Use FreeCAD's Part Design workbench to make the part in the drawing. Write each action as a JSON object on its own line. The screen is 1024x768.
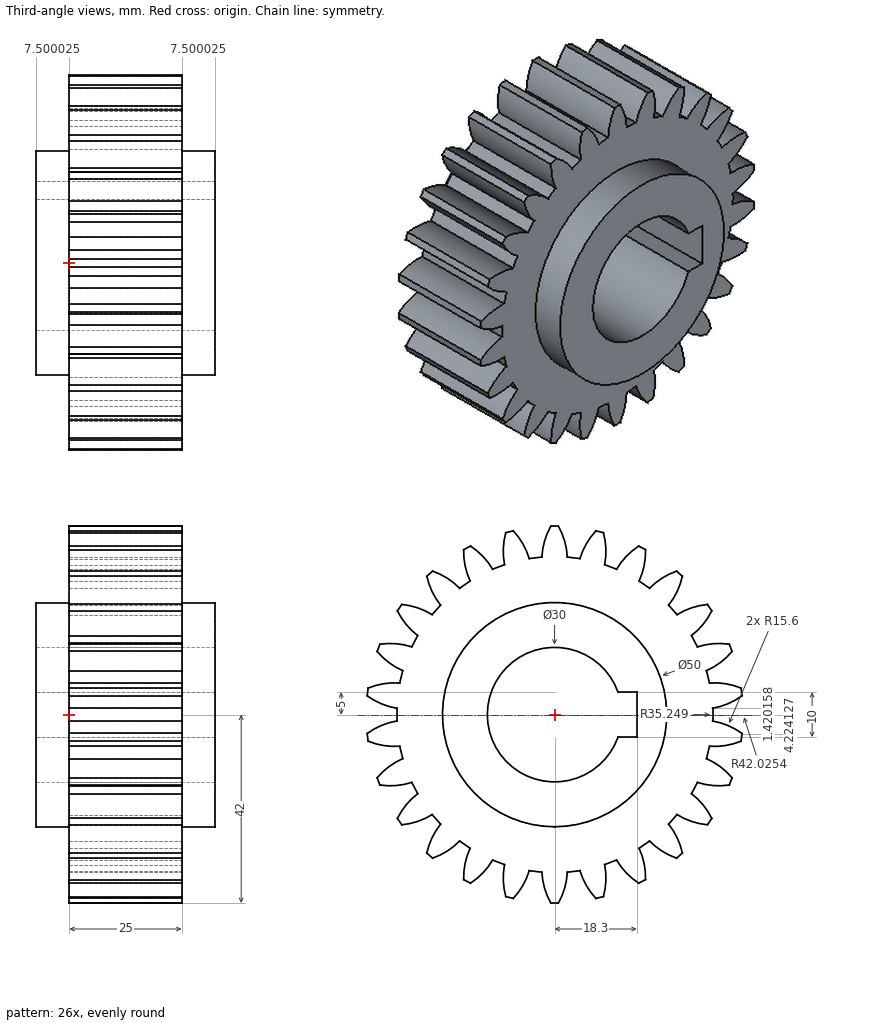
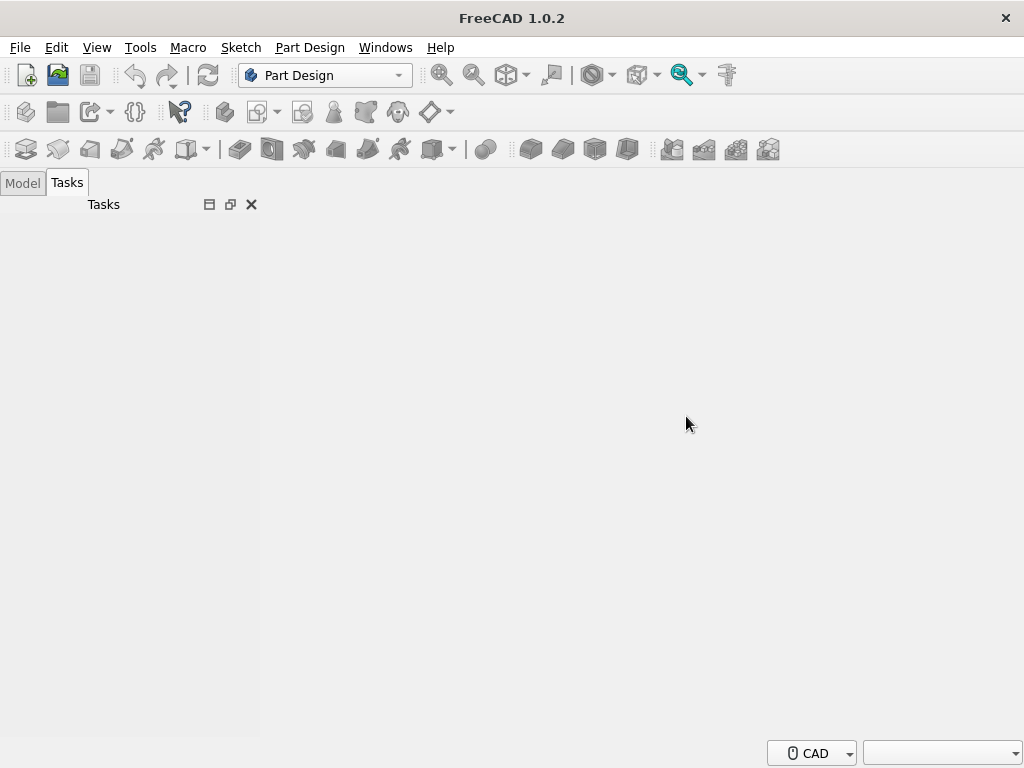
{"action": "left_click", "coordinate": [26, 76]}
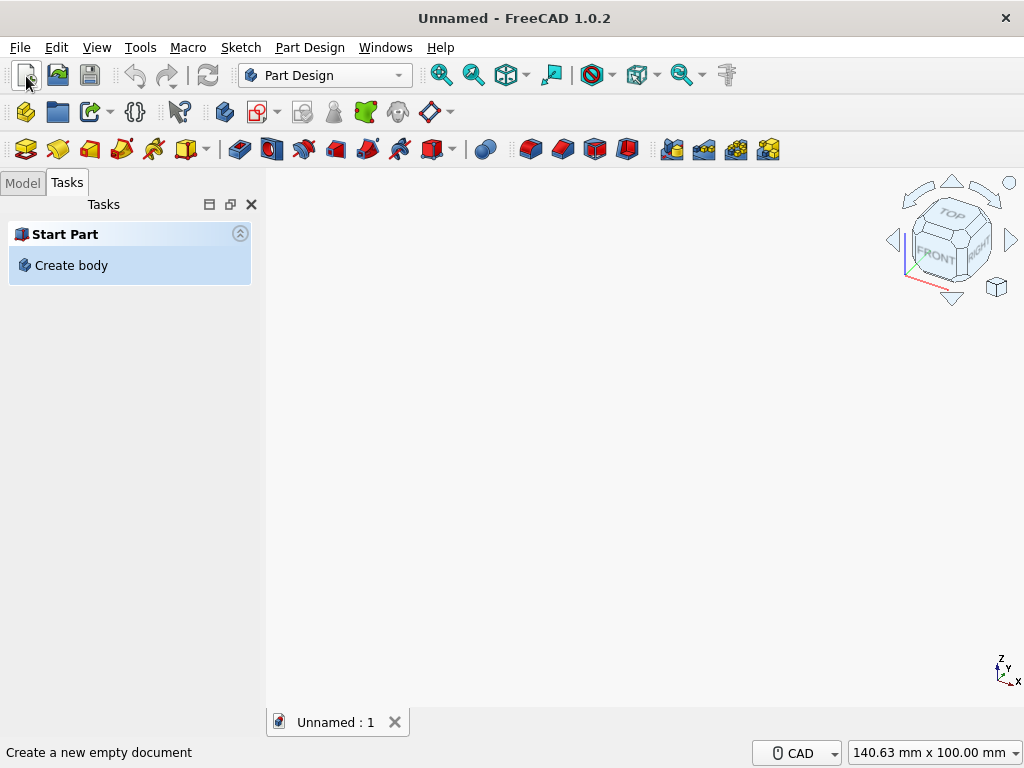
{"action": "left_click", "coordinate": [258, 112]}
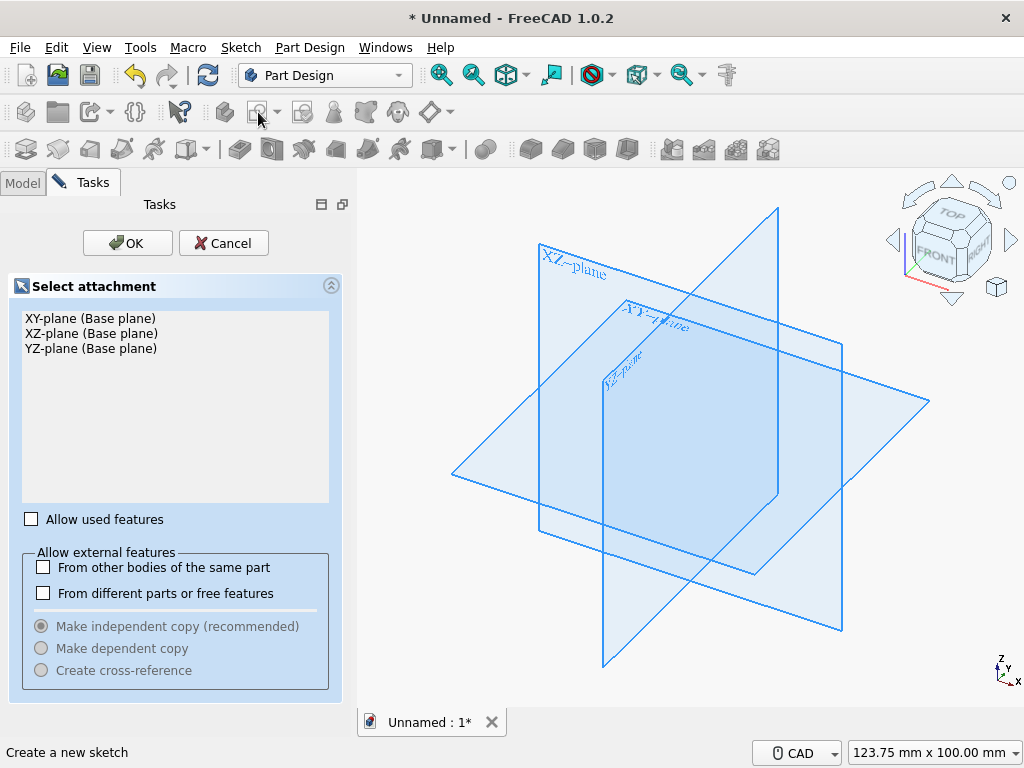
{"action": "left_click", "coordinate": [82, 334]}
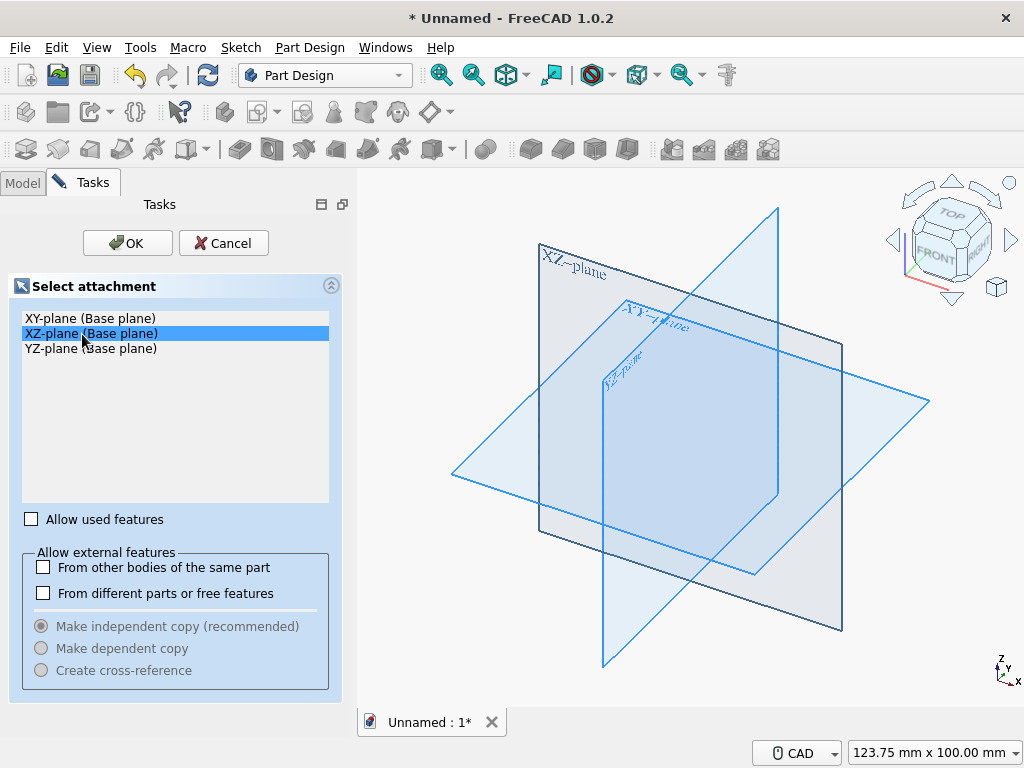
{"action": "left_click", "coordinate": [128, 243]}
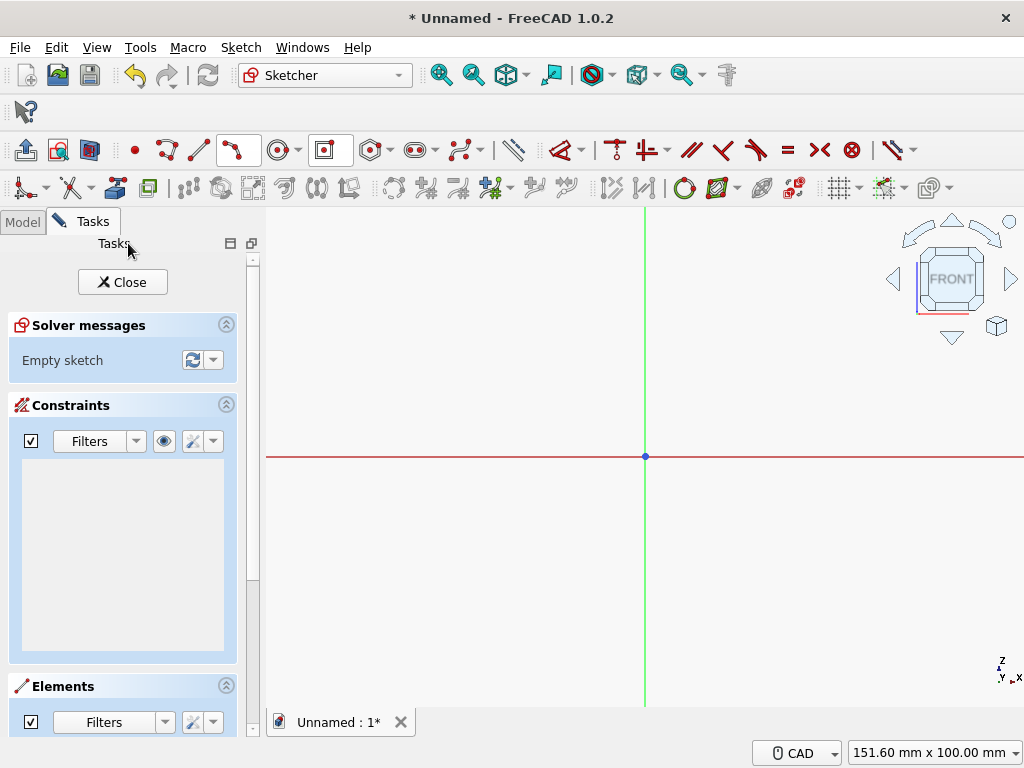
{"action": "scroll", "coordinate": [294, 235], "scroll_direction": "down", "scroll_amount": 1}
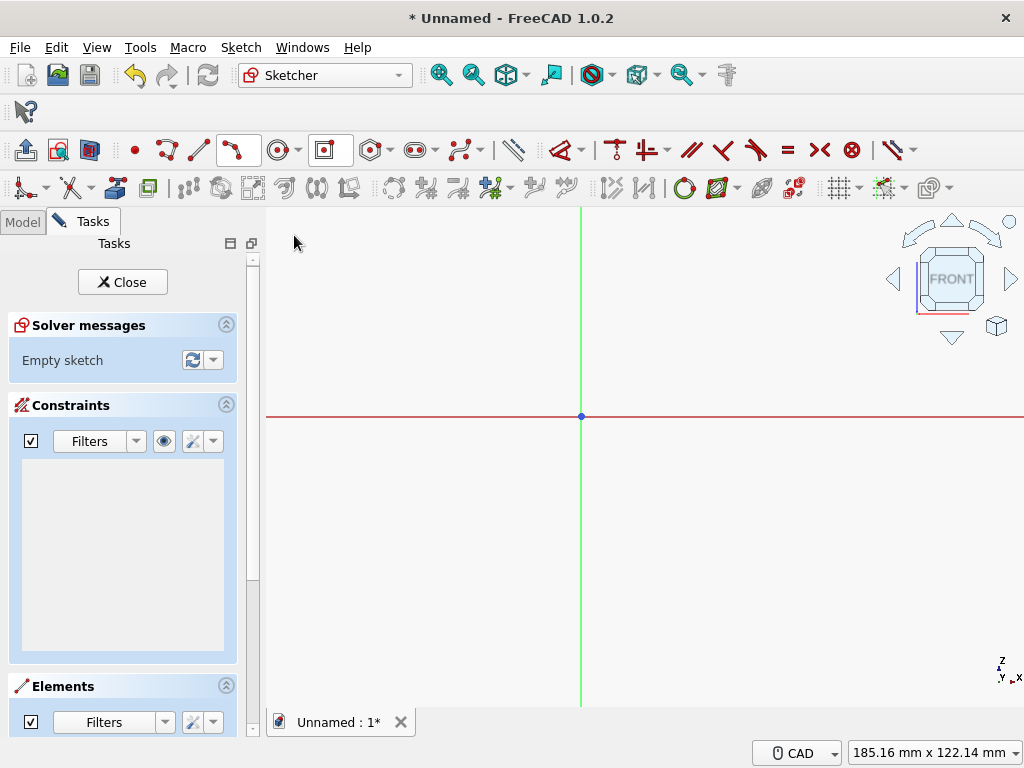
{"action": "scroll", "coordinate": [701, 558], "scroll_direction": "up", "scroll_amount": 3}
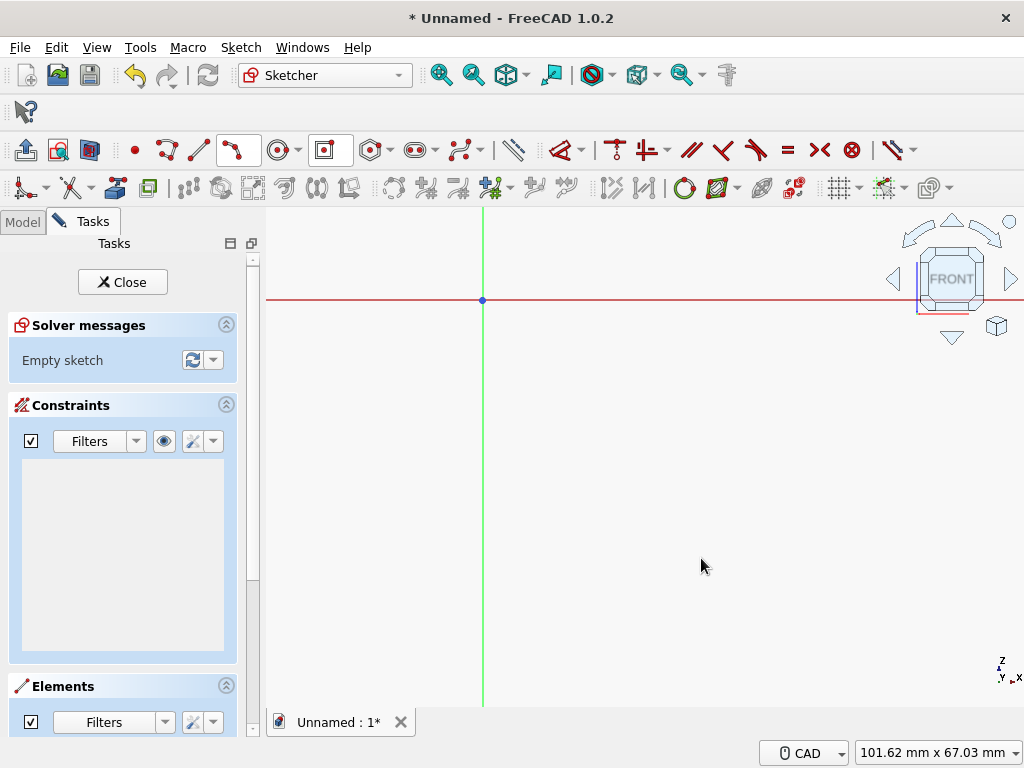
{"action": "left_click", "coordinate": [348, 150]}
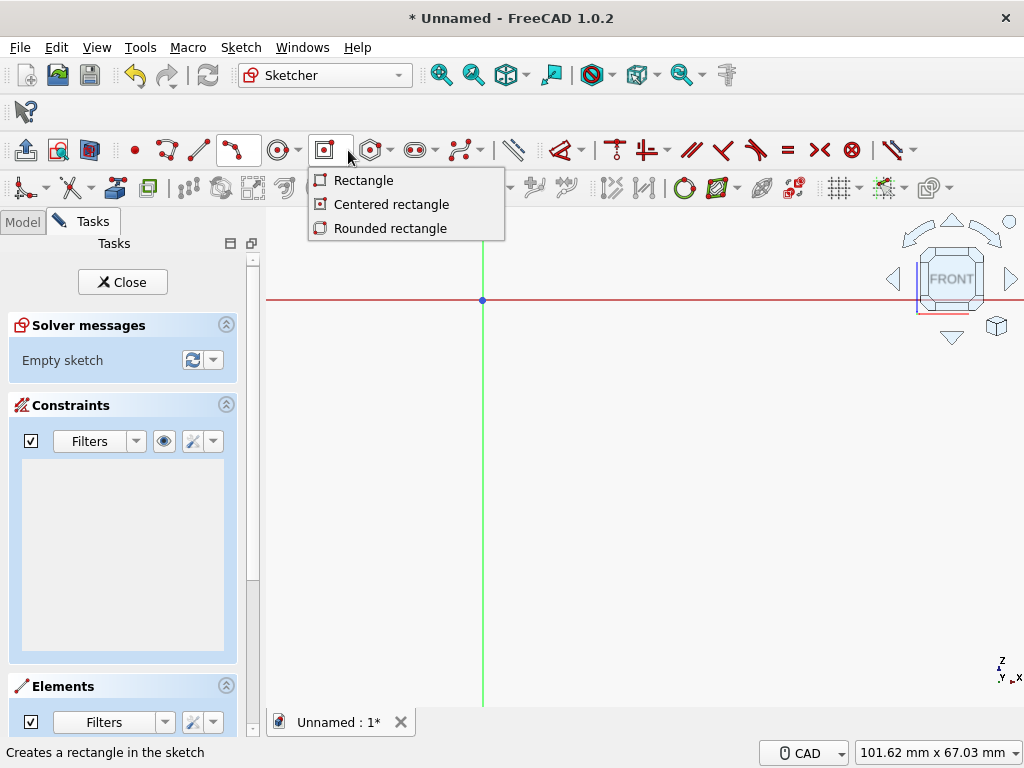
{"action": "left_click", "coordinate": [406, 180]}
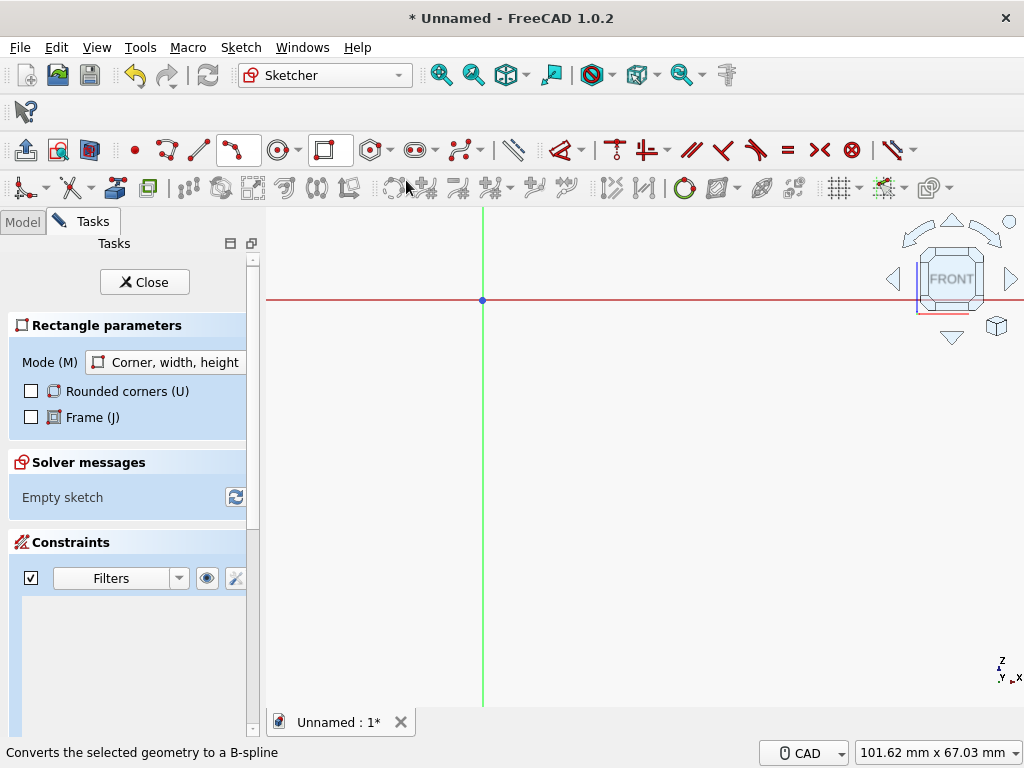
{"action": "left_click", "coordinate": [483, 300]}
{"action": "mouse_move", "coordinate": [669, 613]}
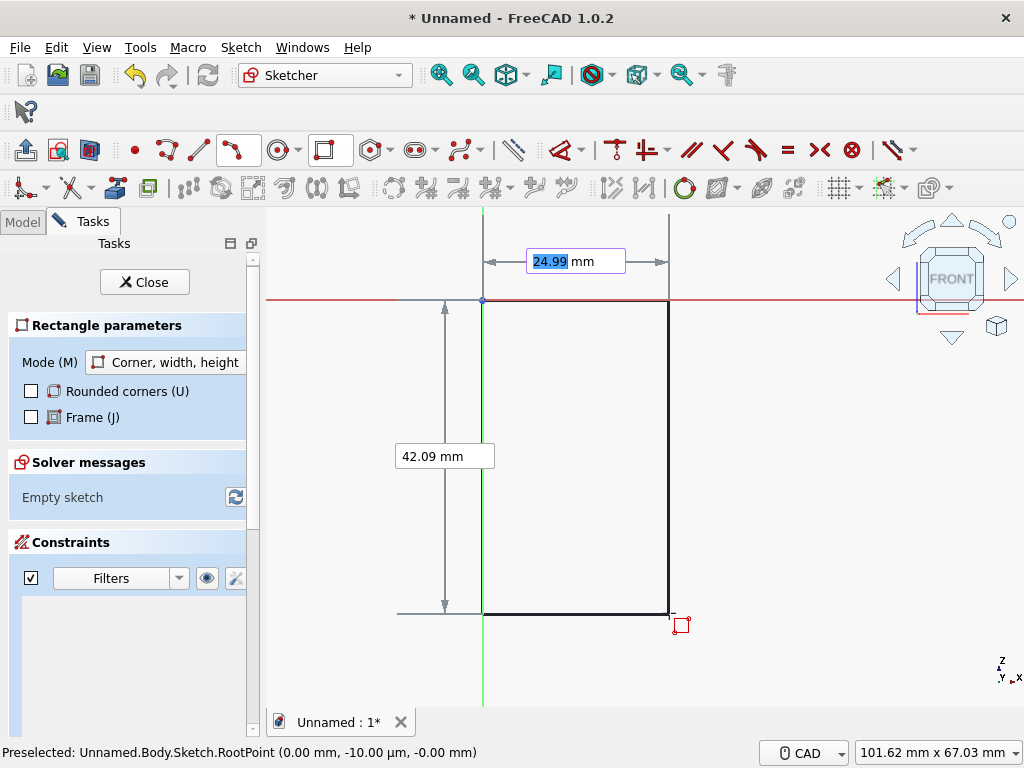
{"action": "type", "text": "25"}
{"action": "key", "text": "Tab"}
{"action": "type", "text": "42"}
{"action": "key", "text": "Return"}
{"action": "key", "text": "Escape"}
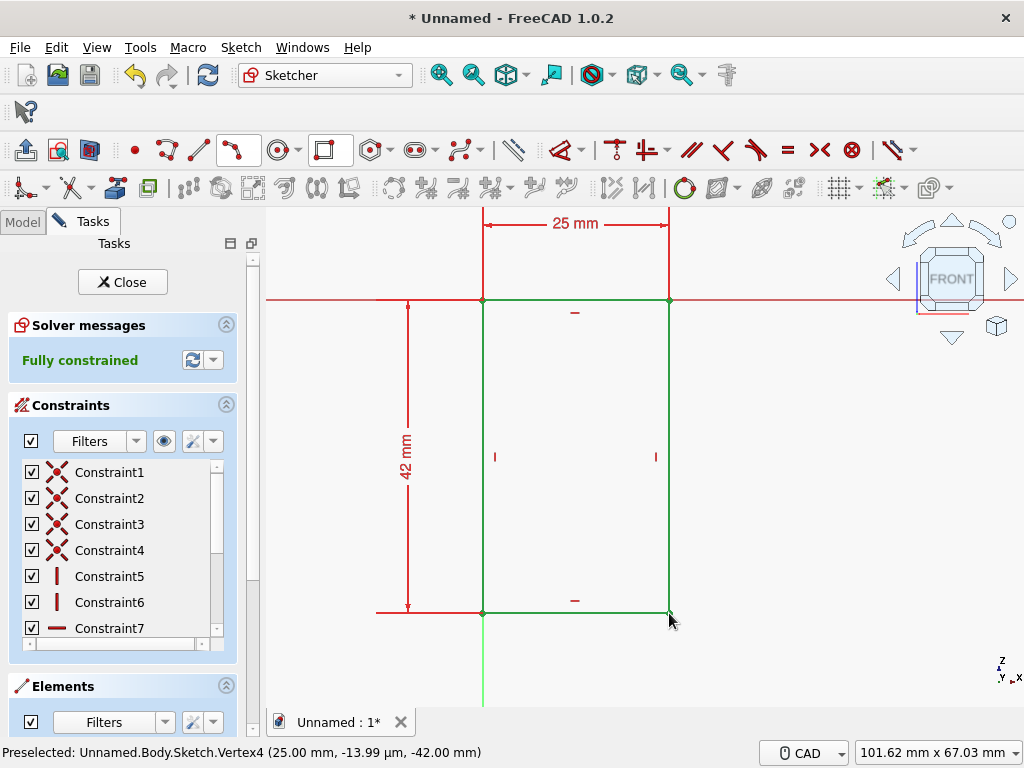
{"action": "left_click", "coordinate": [123, 282]}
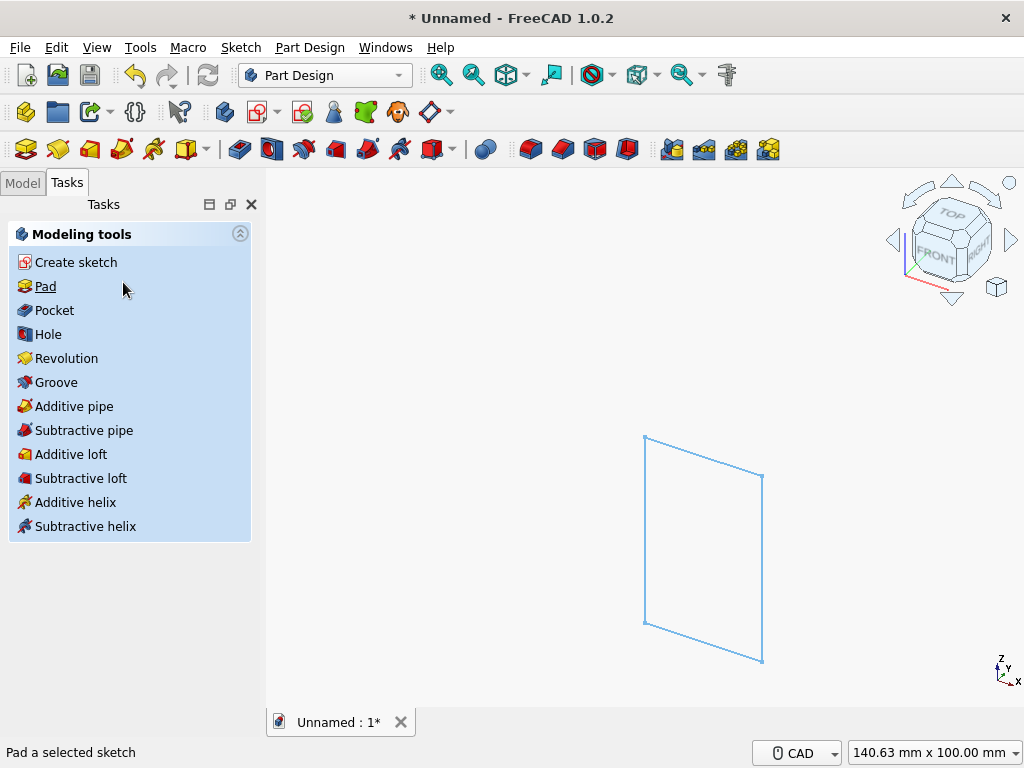
{"action": "left_click", "coordinate": [58, 150]}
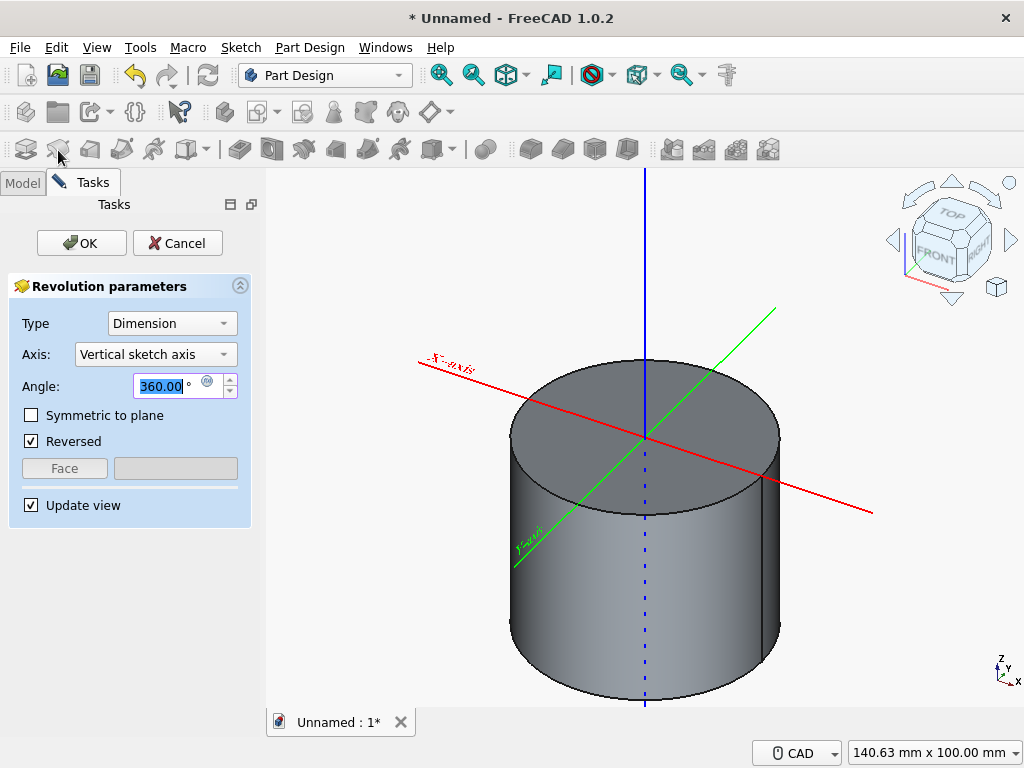
{"action": "left_click", "coordinate": [156, 354]}